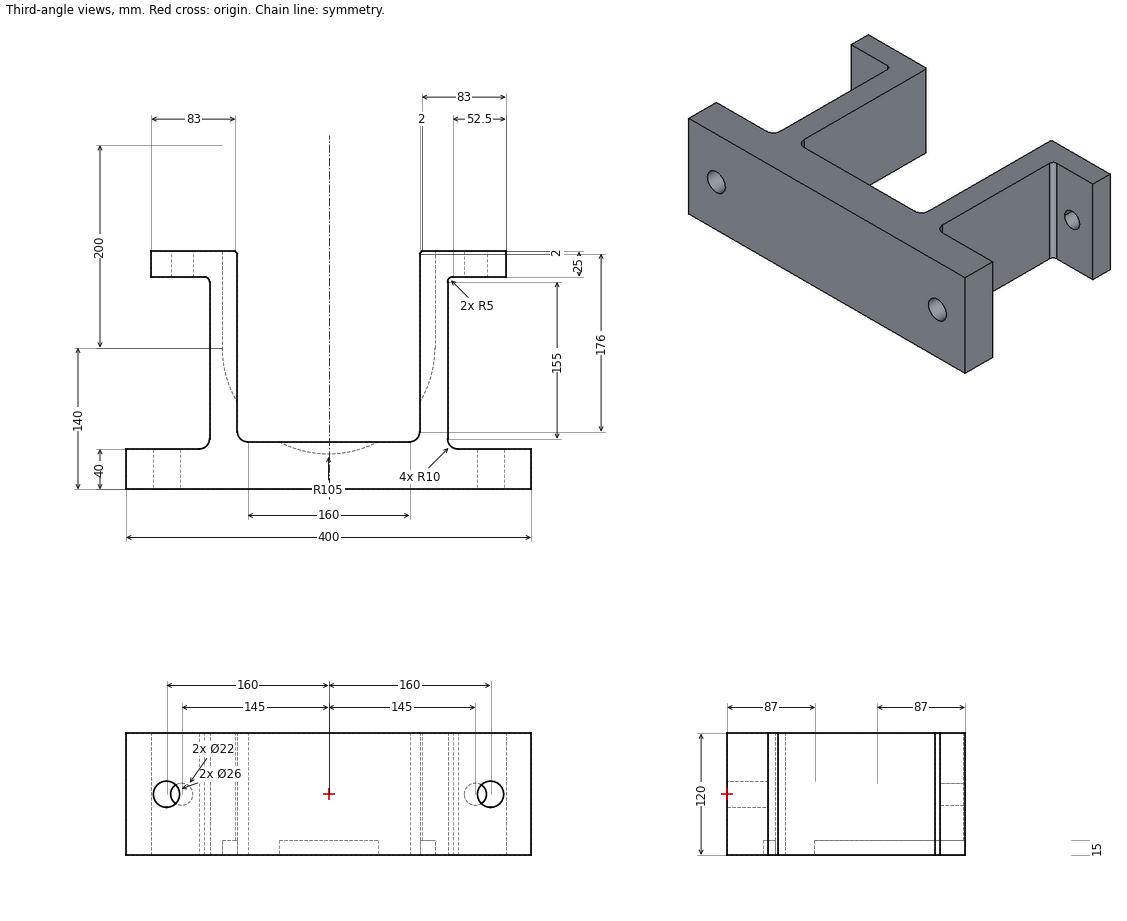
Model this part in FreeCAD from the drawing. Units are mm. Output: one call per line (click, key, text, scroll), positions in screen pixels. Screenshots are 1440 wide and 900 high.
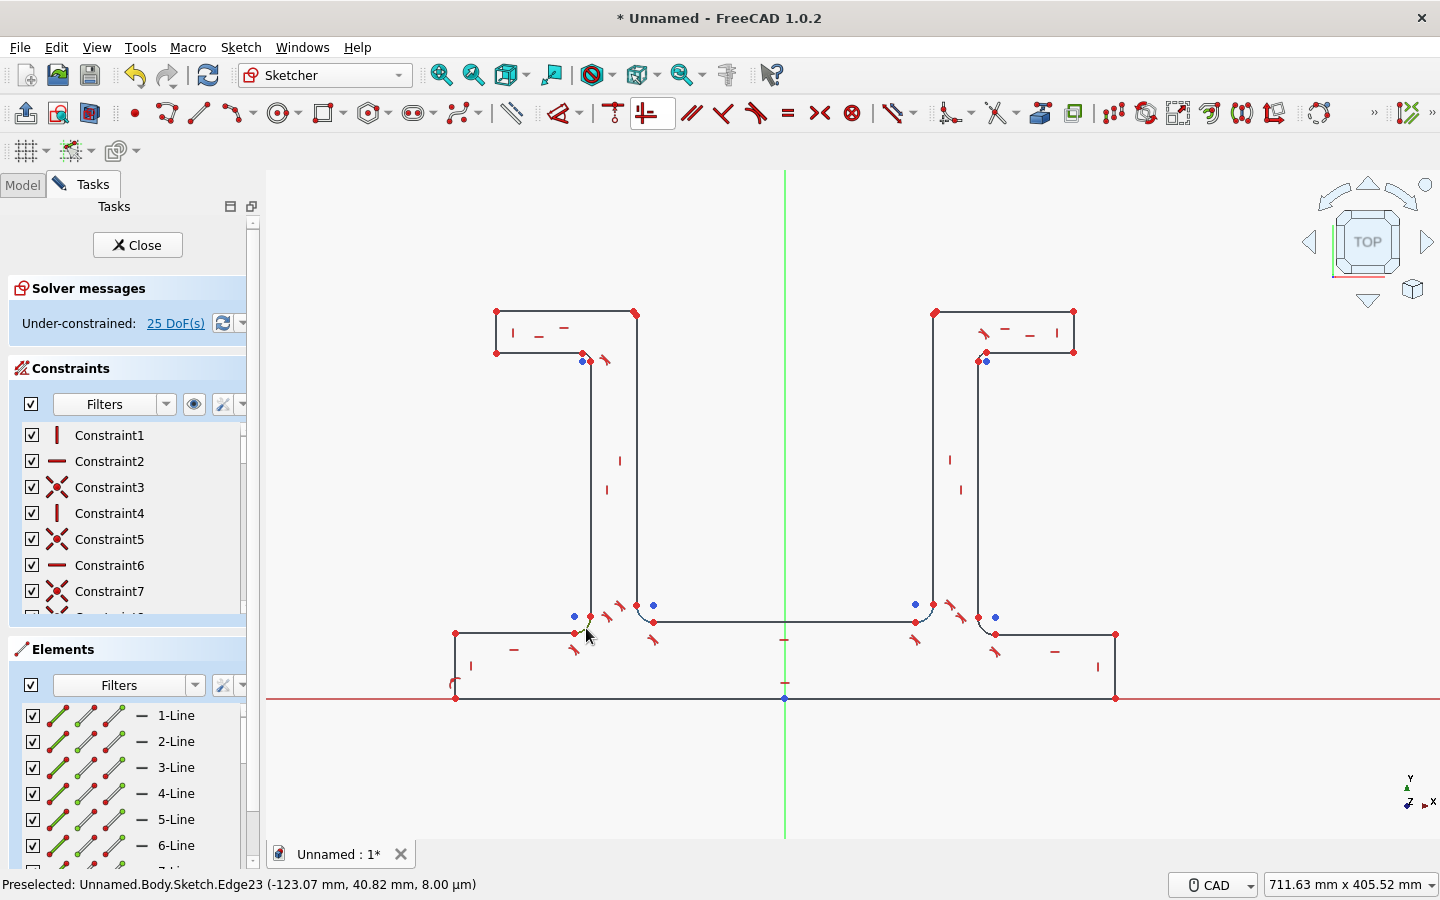
click(983, 630)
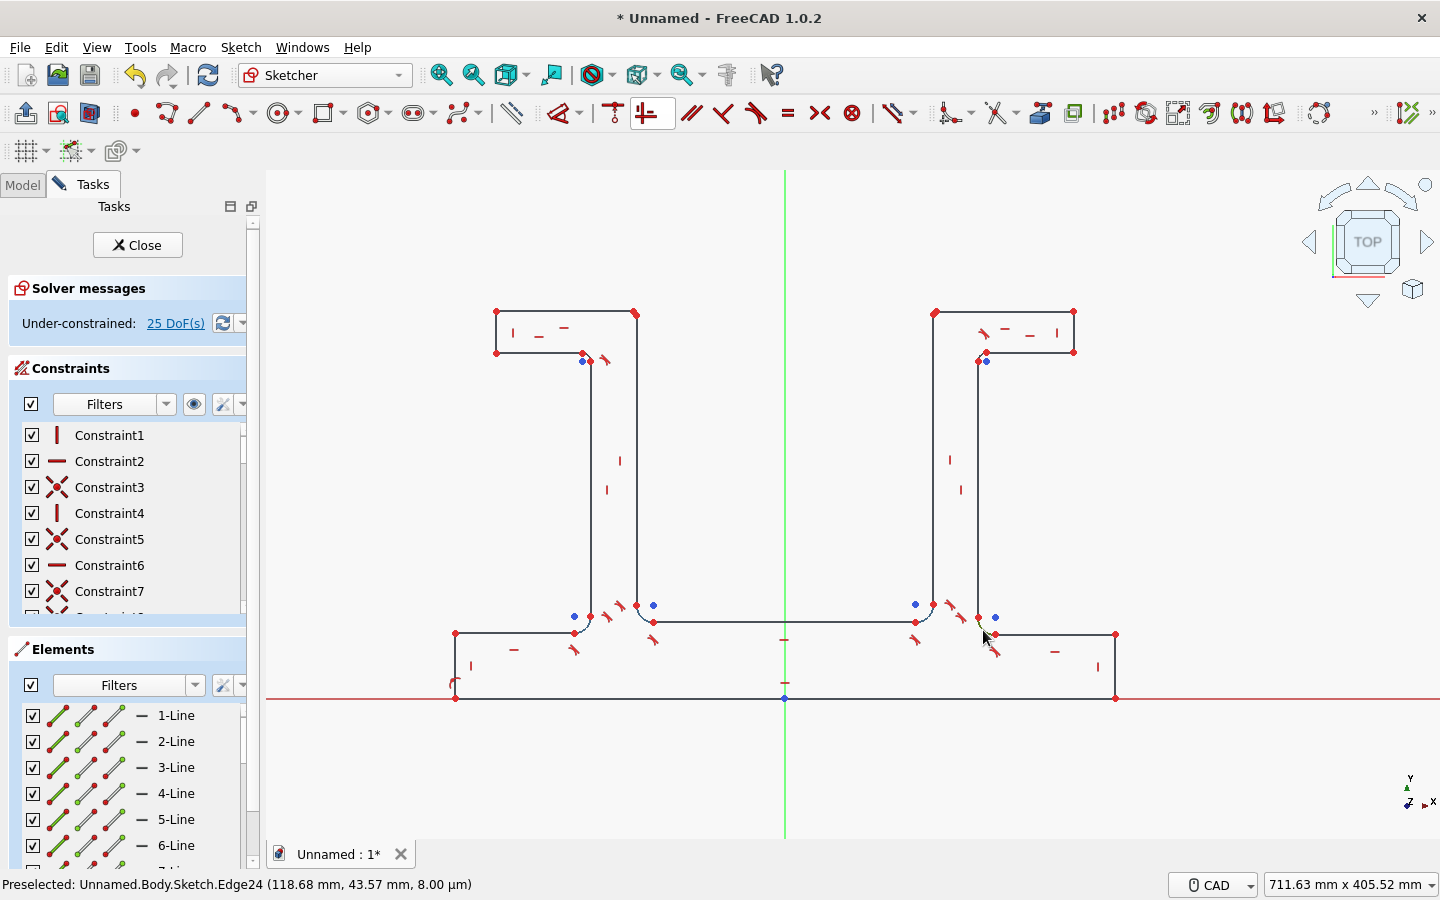
click(788, 114)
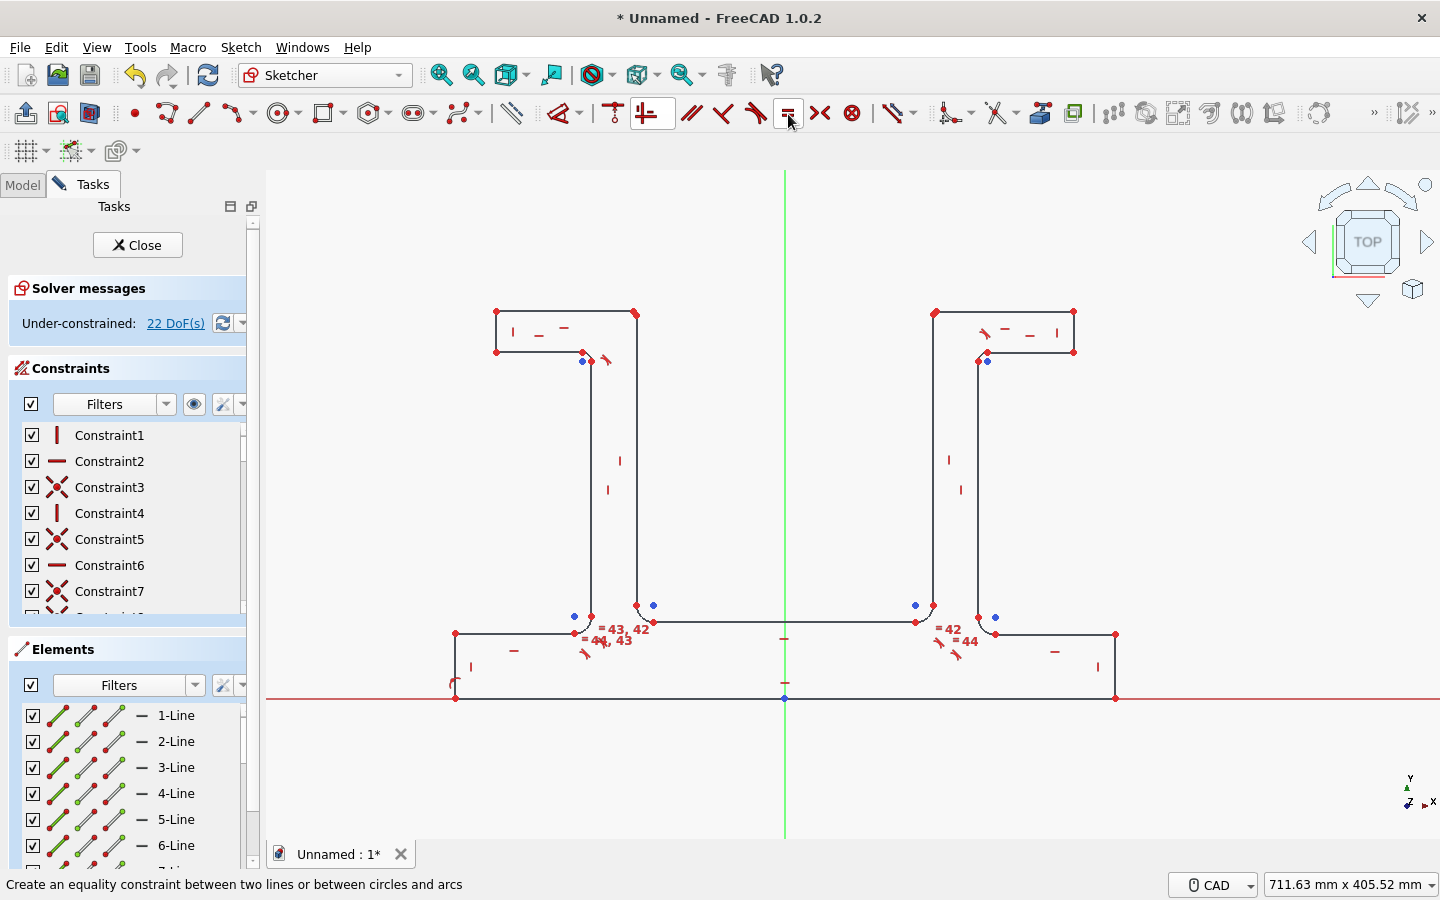
scroll(981, 355, up, 4)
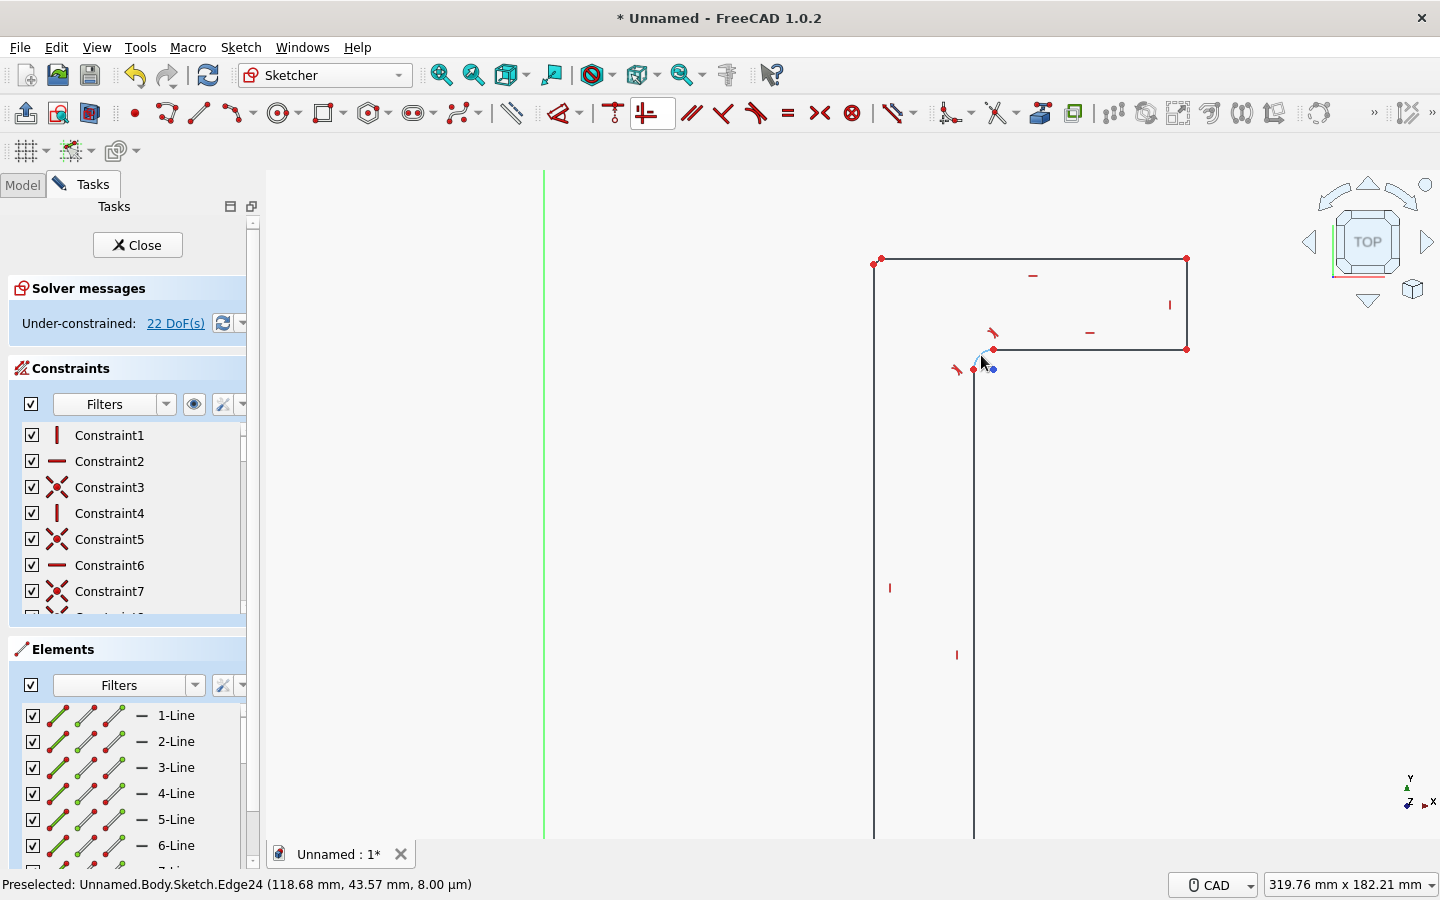
click(980, 355)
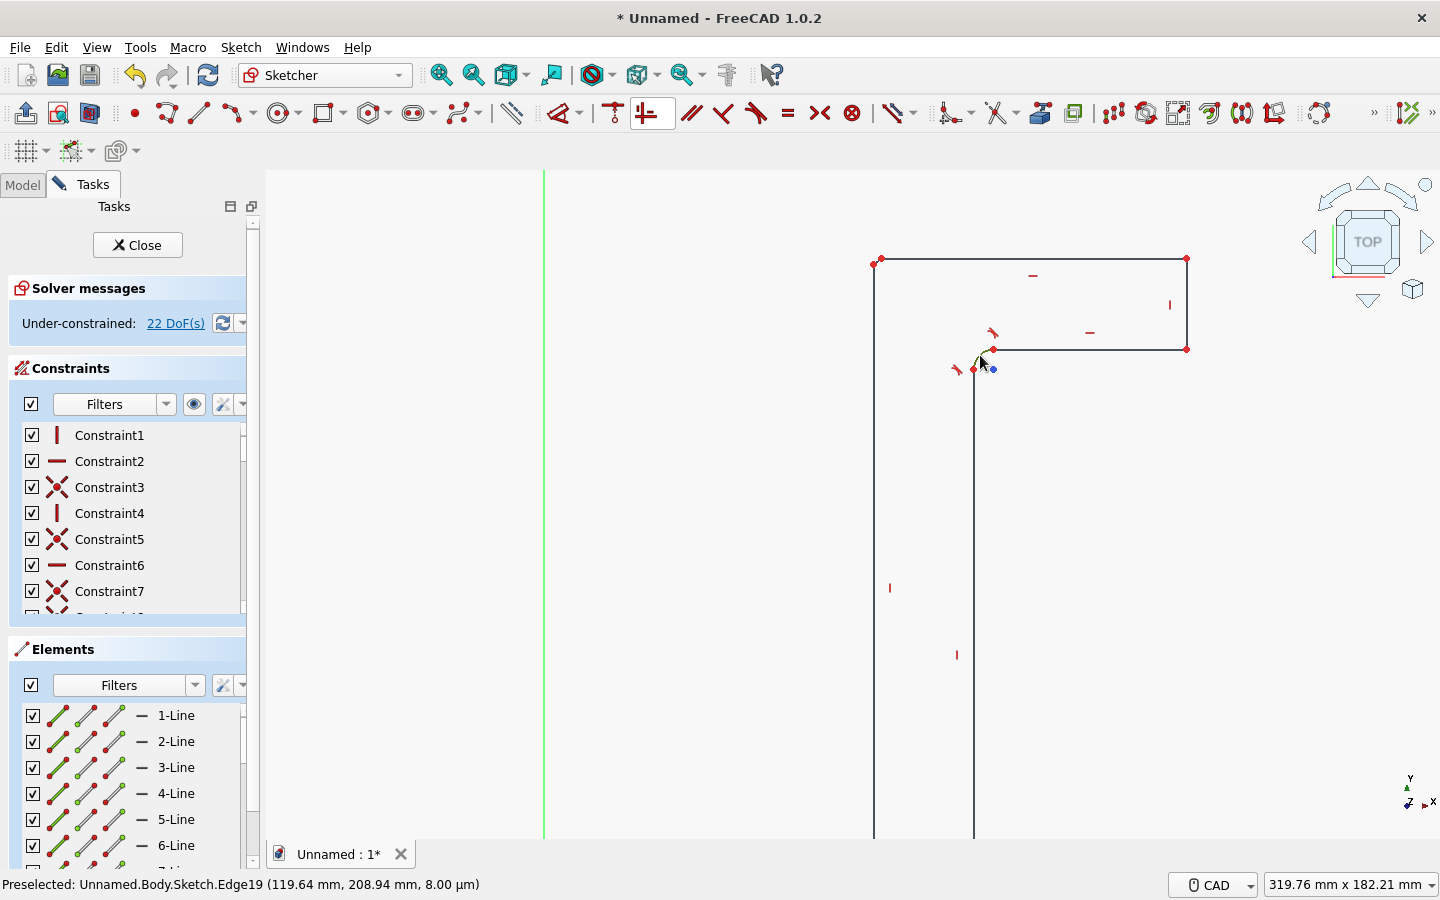
scroll(981, 355, down, 4)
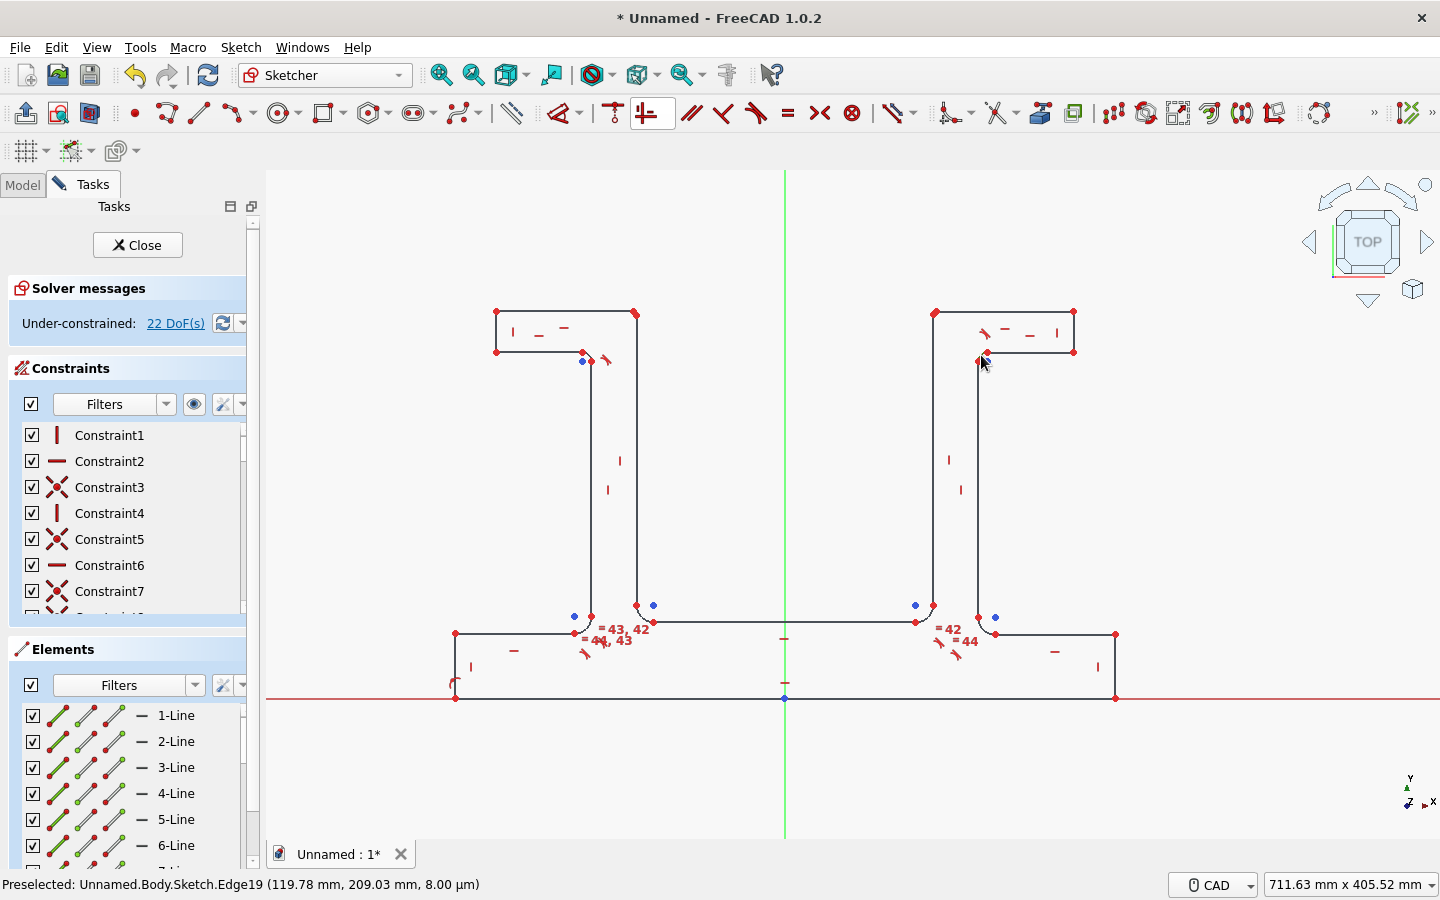
scroll(591, 357, up, 6)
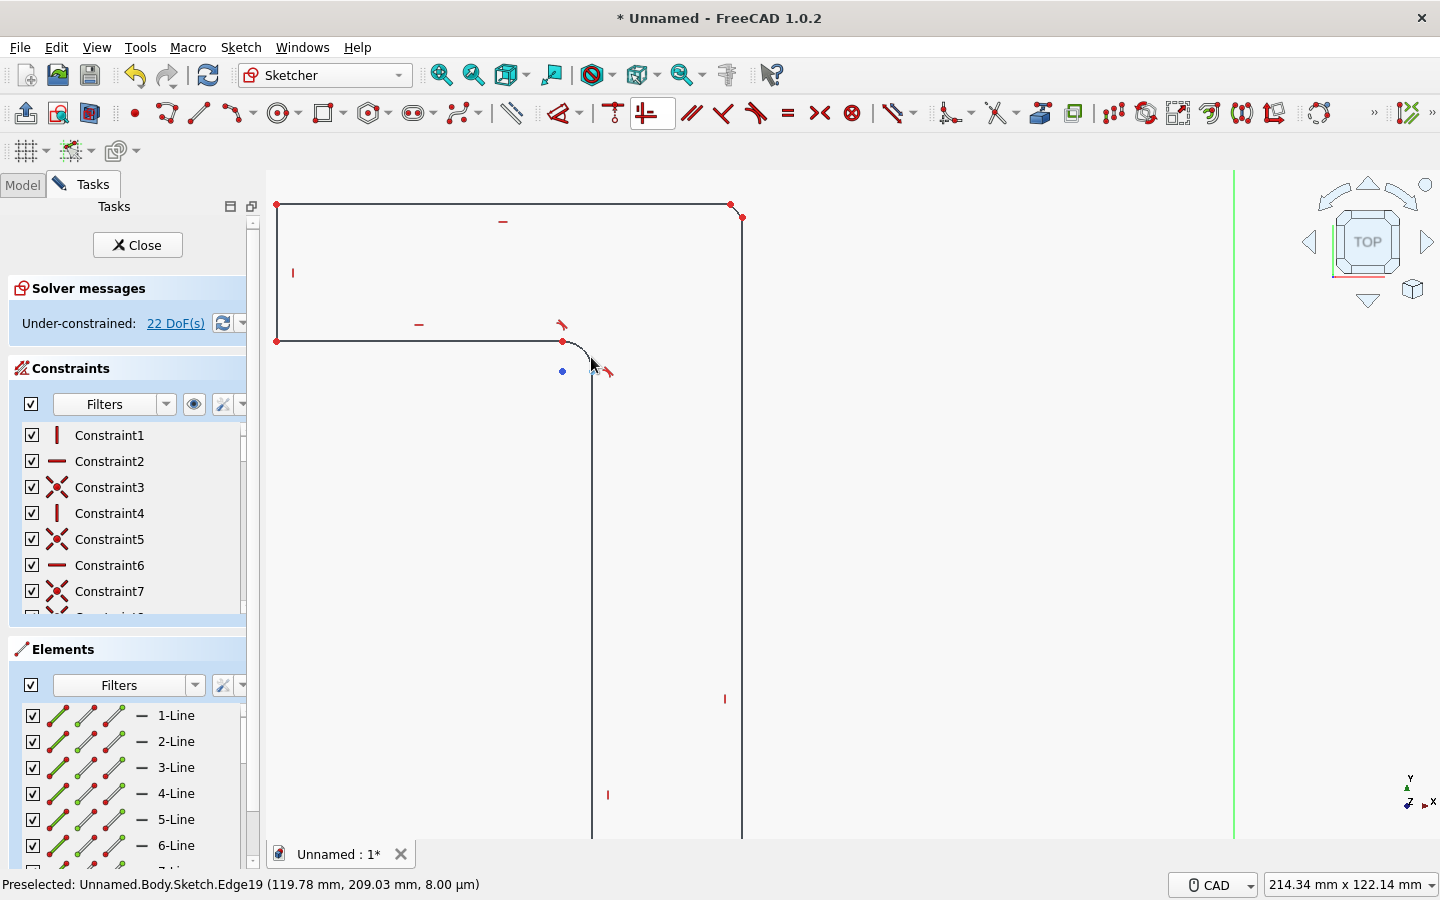
click(589, 358)